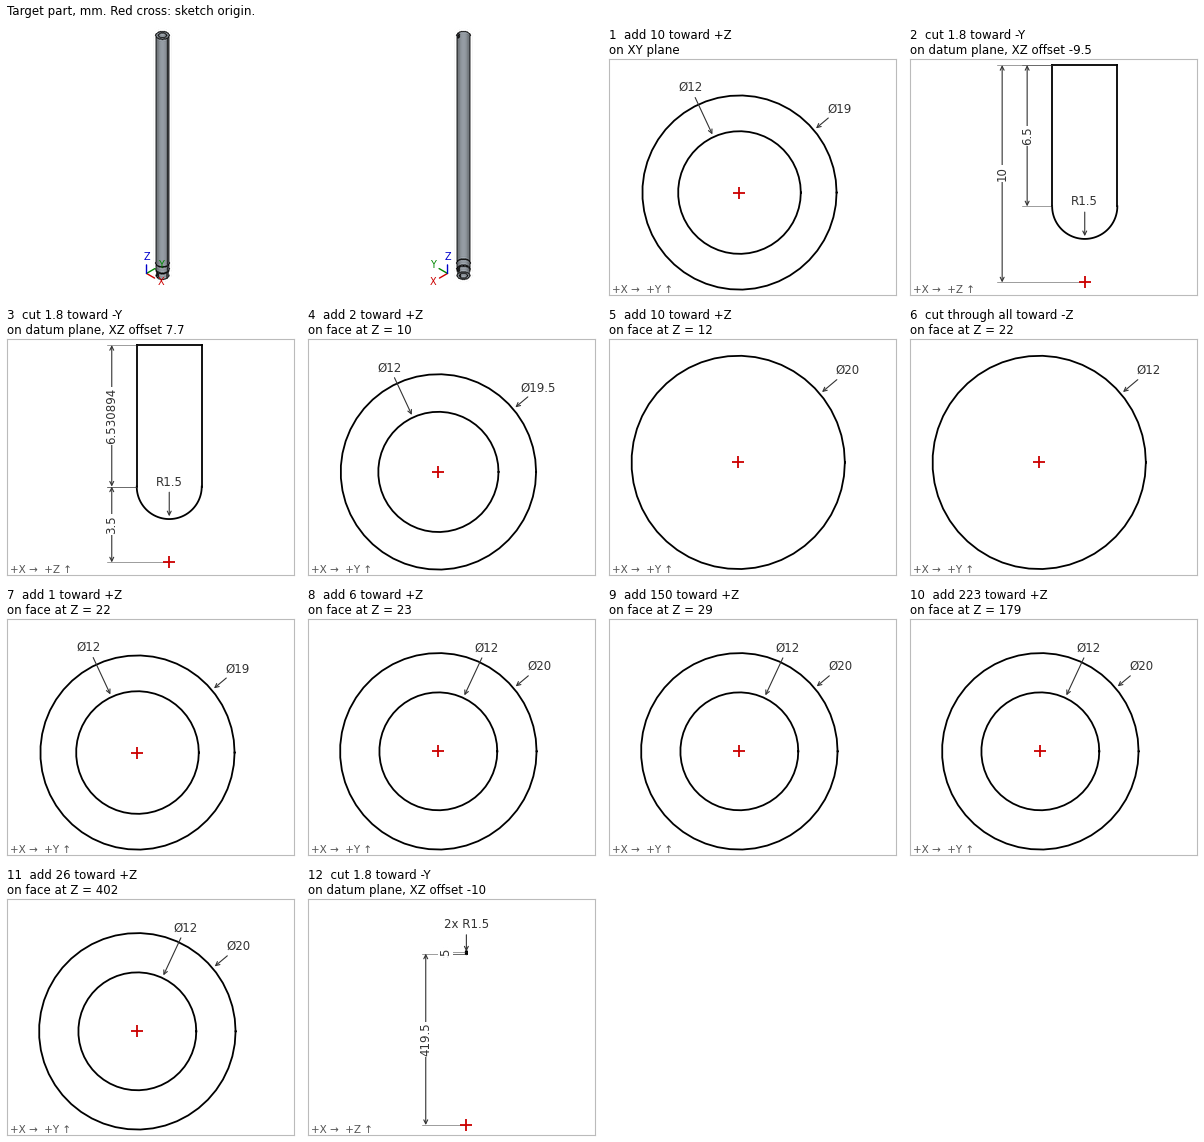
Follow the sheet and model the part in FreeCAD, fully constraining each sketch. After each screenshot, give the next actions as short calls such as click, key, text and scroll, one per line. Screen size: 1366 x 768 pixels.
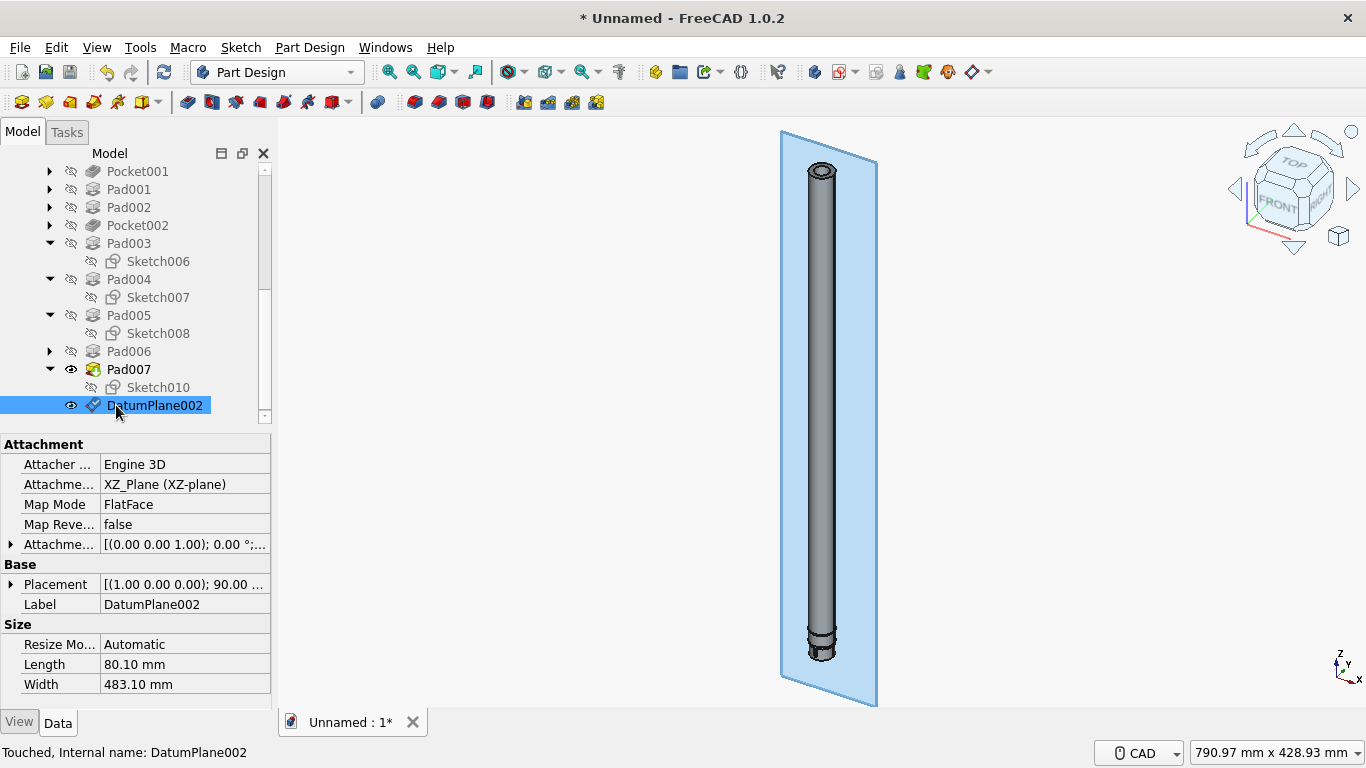
click(840, 72)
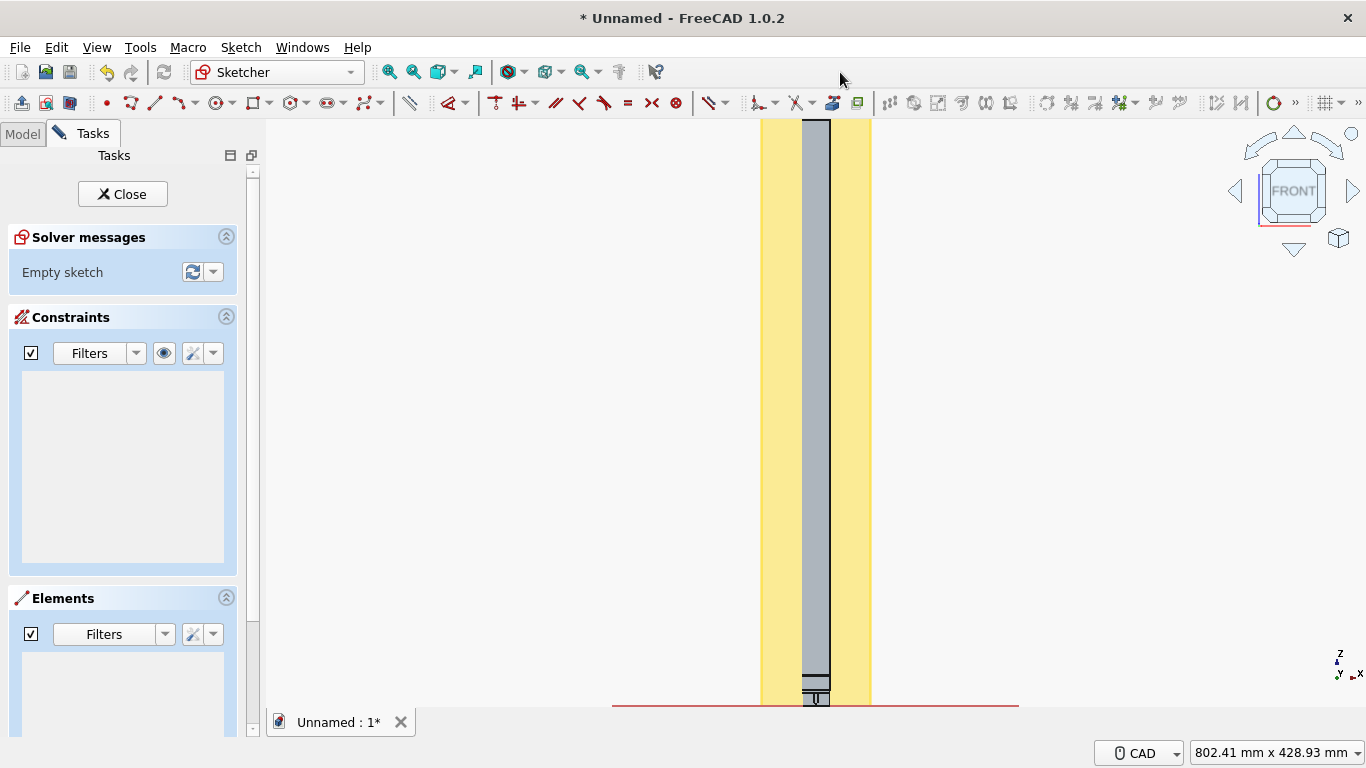
click(70, 104)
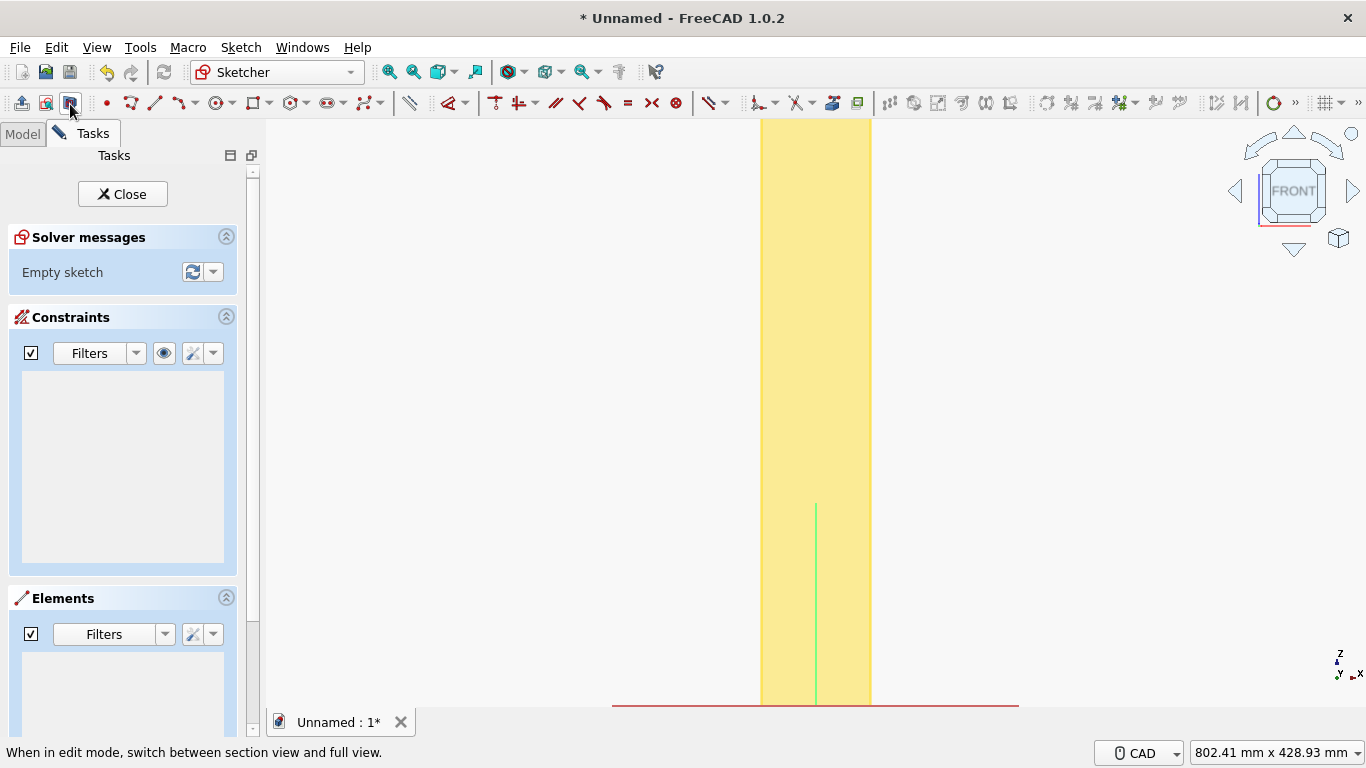
scroll(748, 413, down, 5)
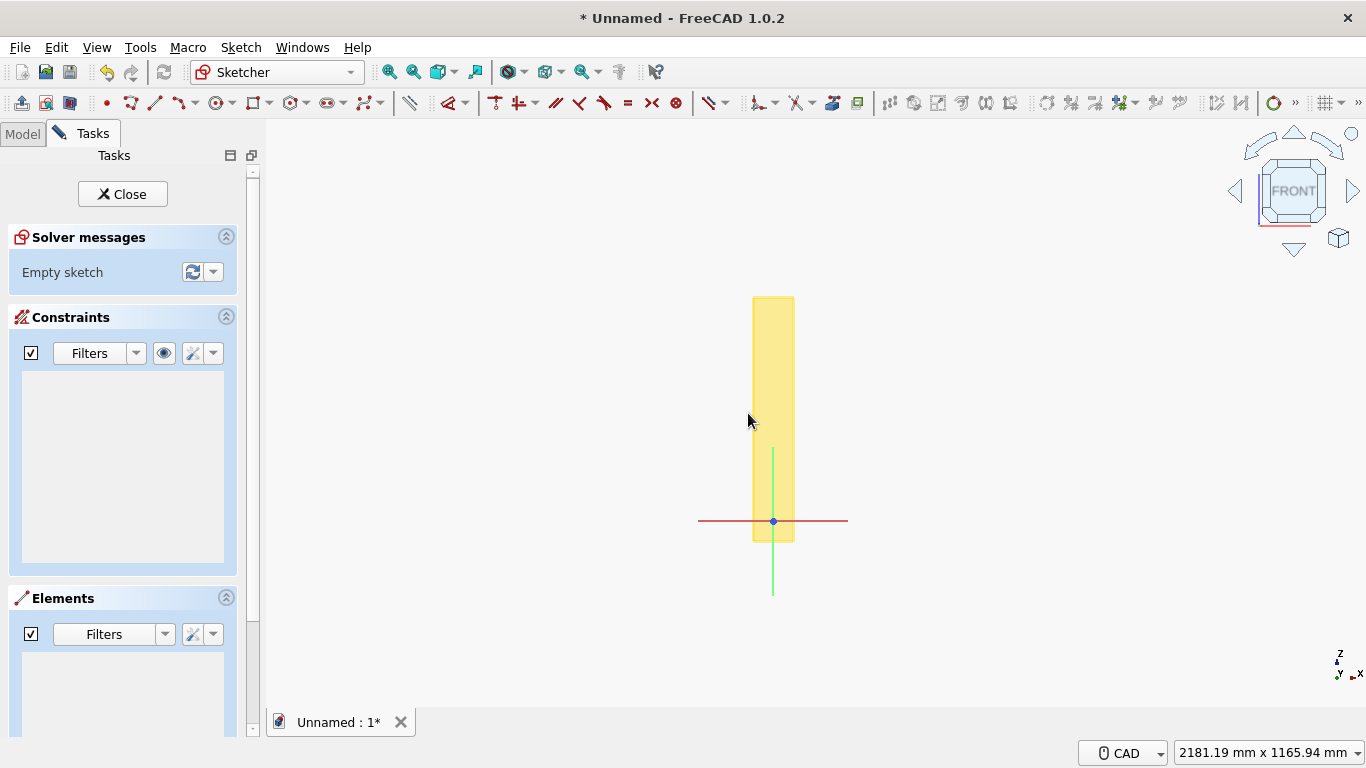
scroll(775, 303, up, 15)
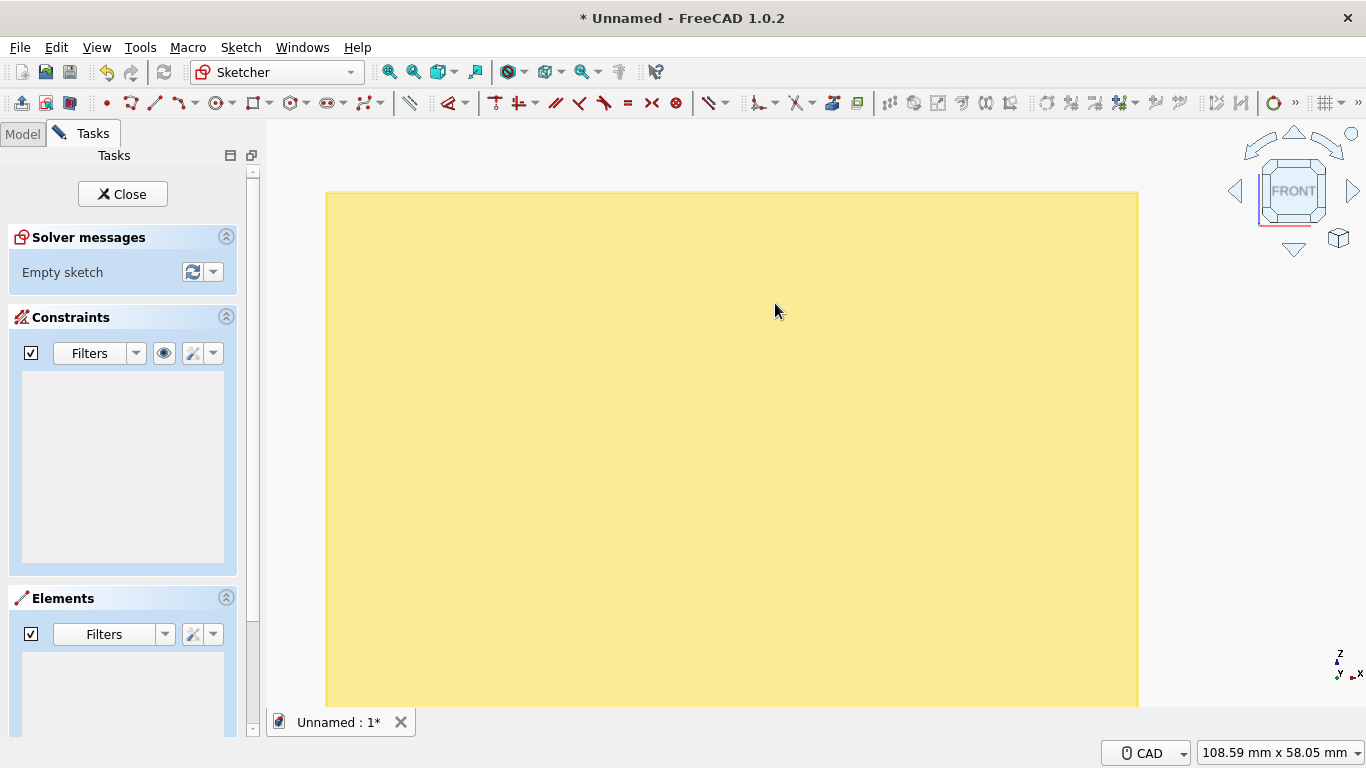
scroll(728, 404, up, 8)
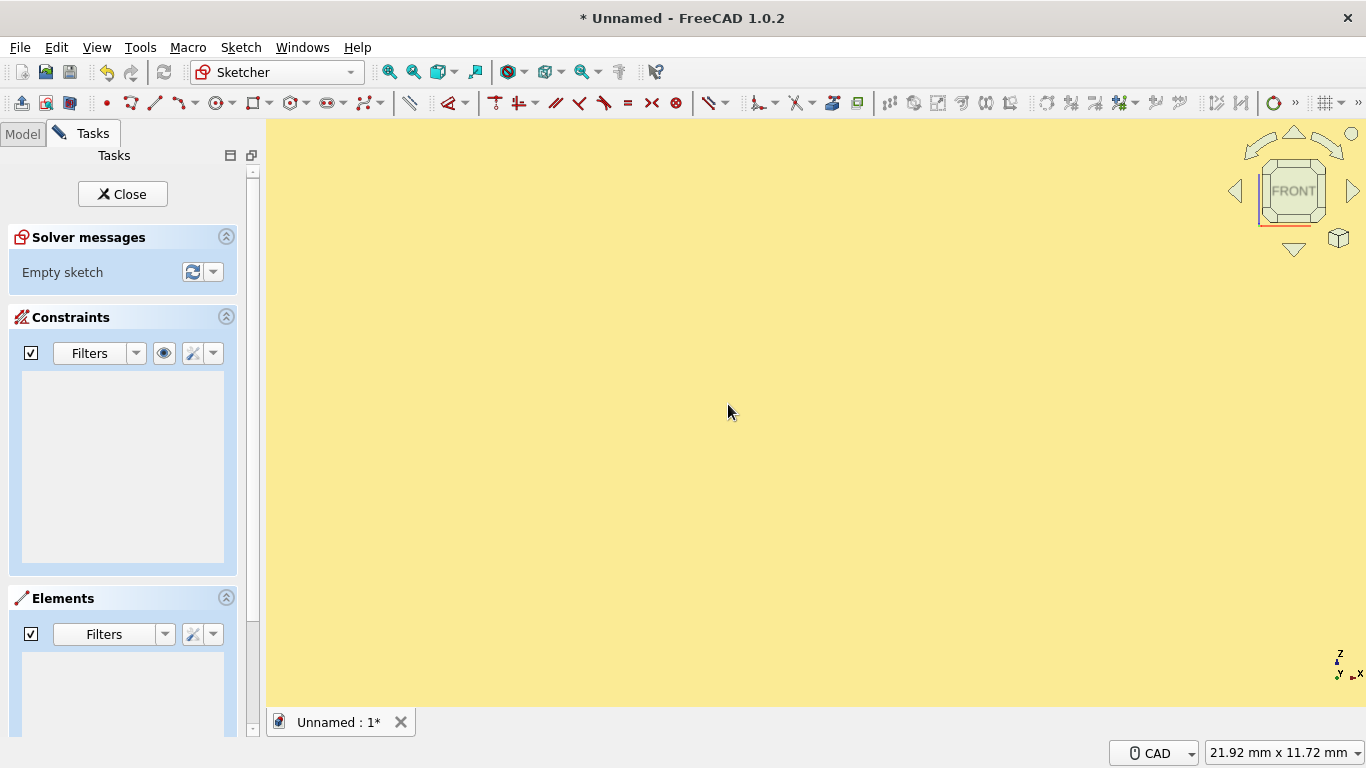
click(328, 104)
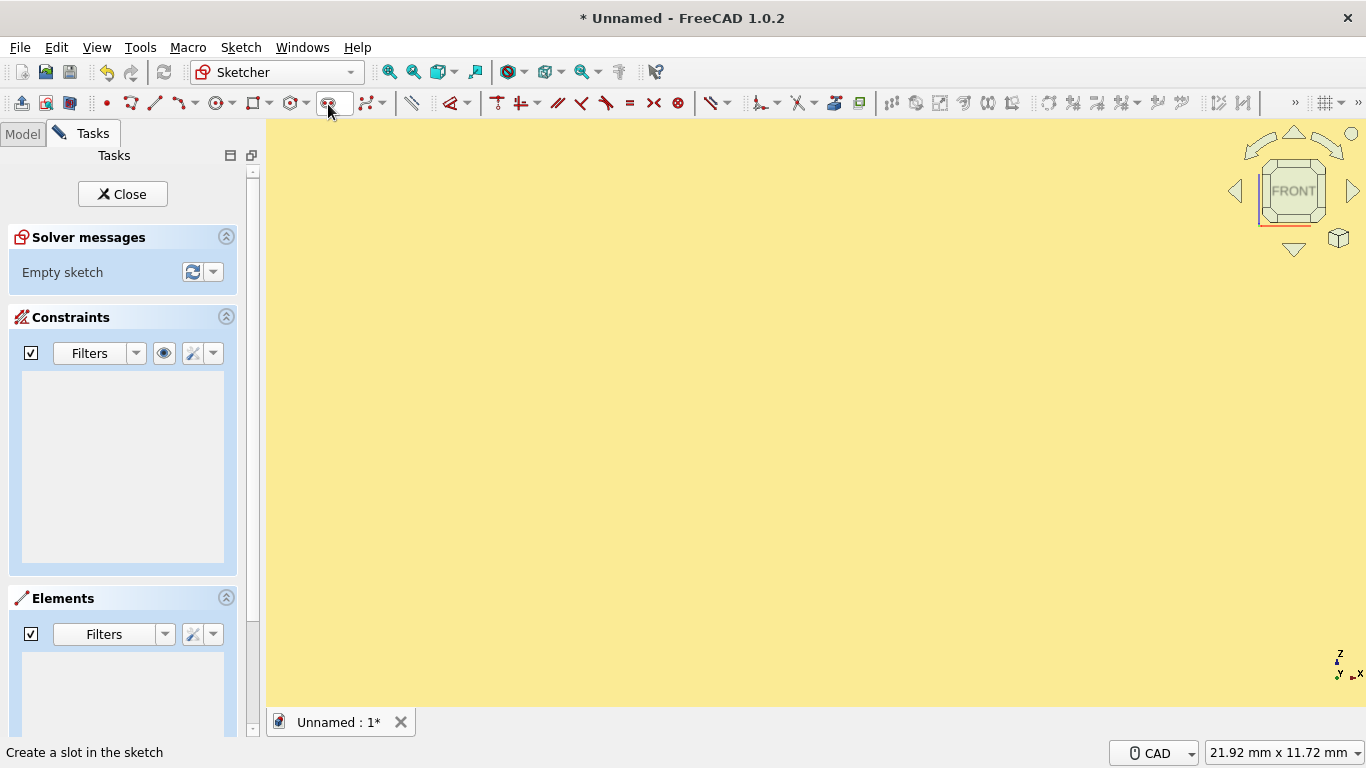
click(746, 537)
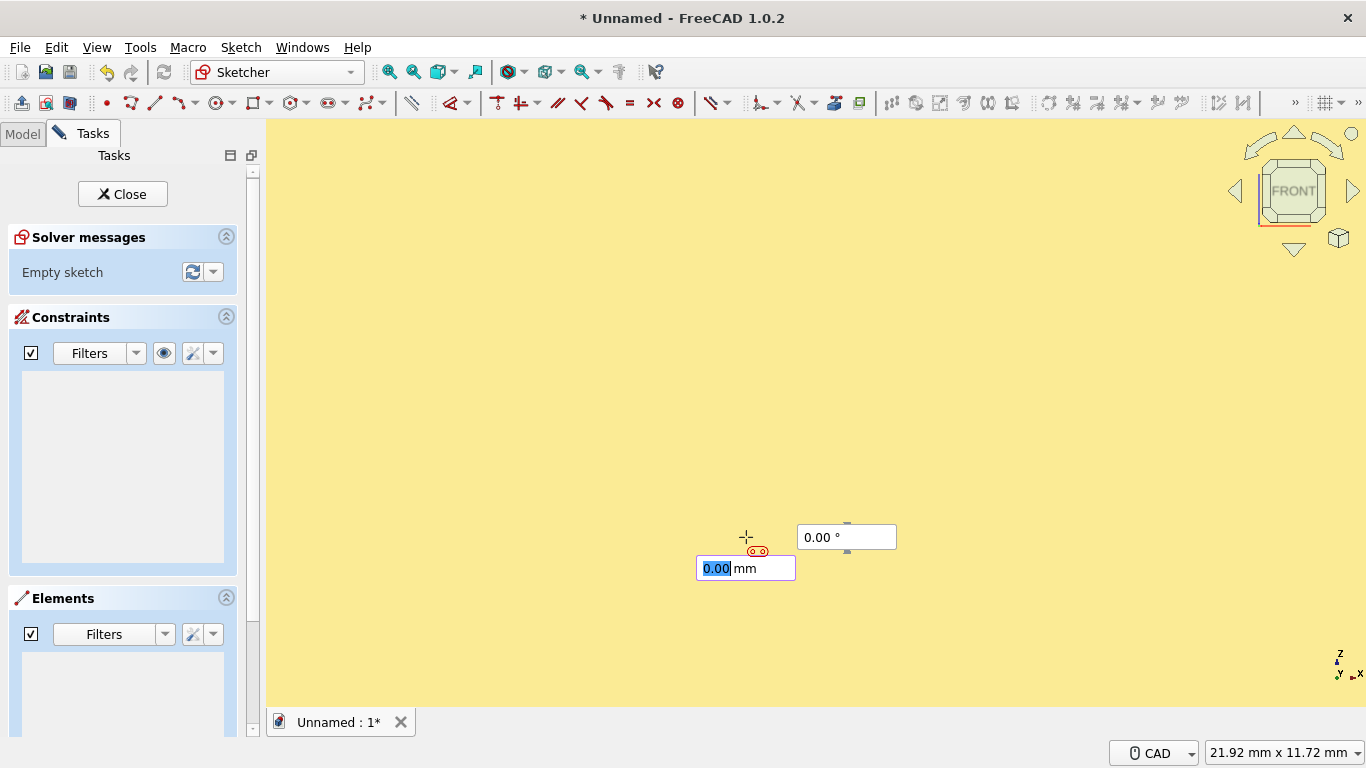
click(755, 286)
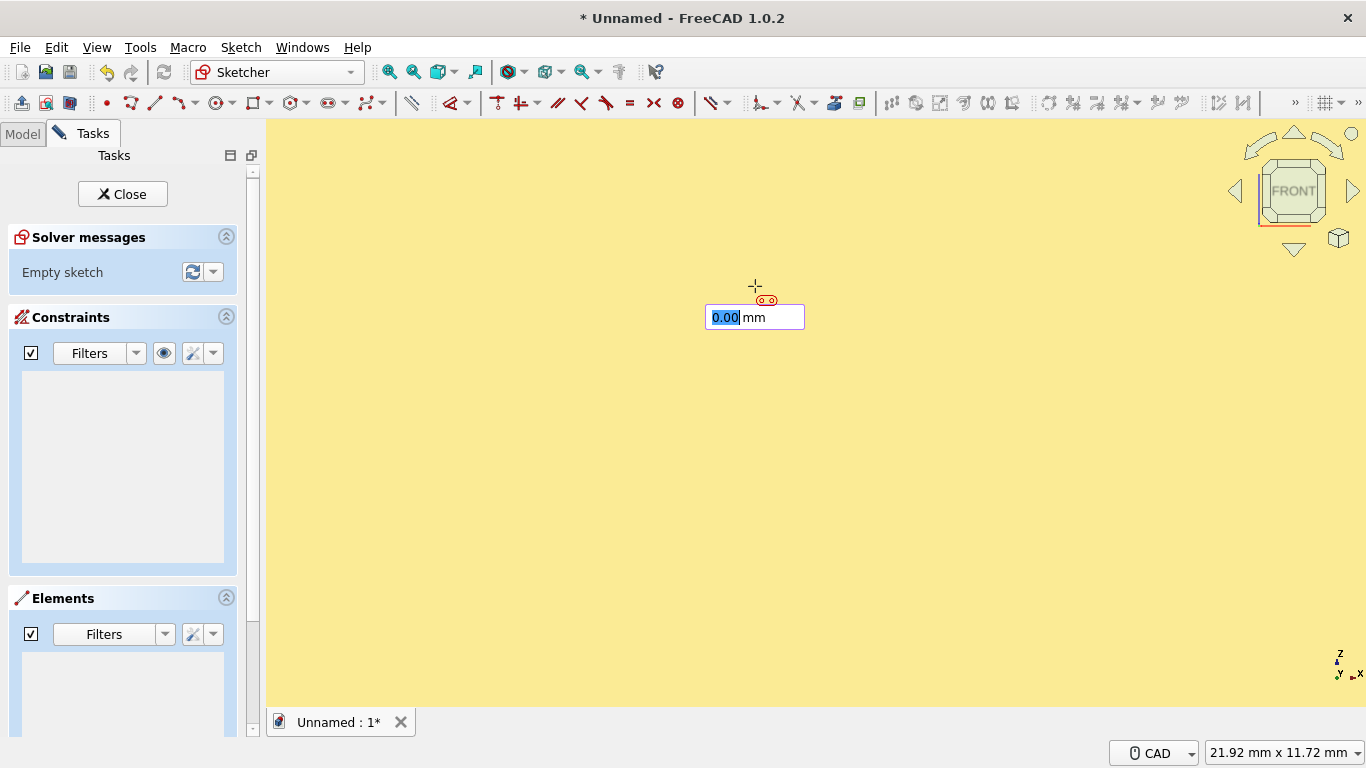
click(821, 411)
key(Escape)